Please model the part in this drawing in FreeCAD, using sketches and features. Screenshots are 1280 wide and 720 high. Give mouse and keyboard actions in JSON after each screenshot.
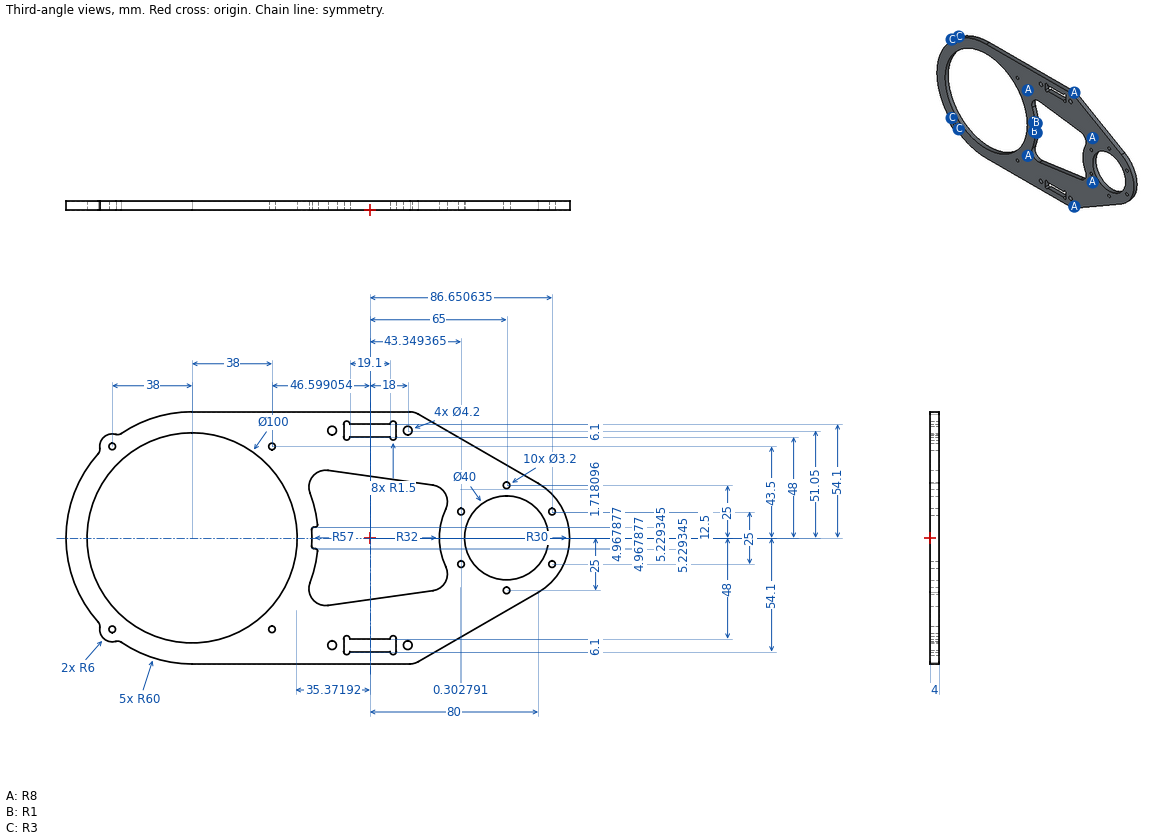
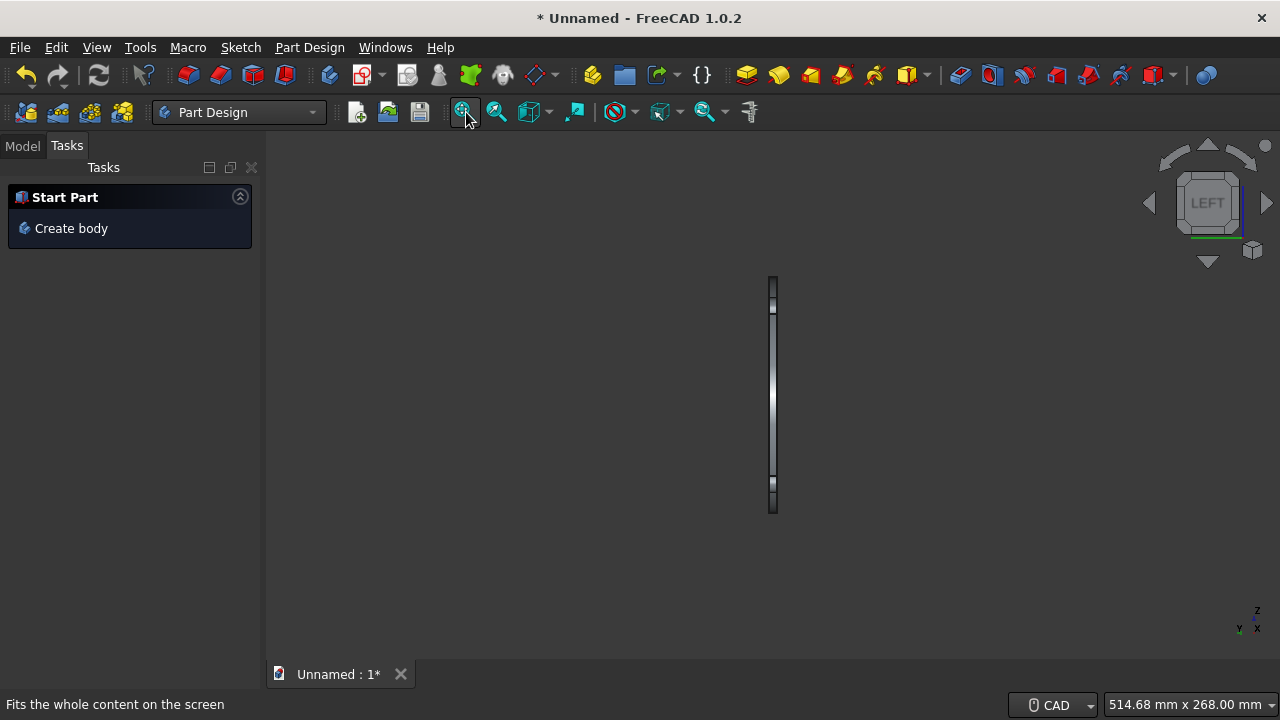
{"action": "scroll", "coordinate": [773, 298], "scroll_direction": "up", "scroll_amount": 9}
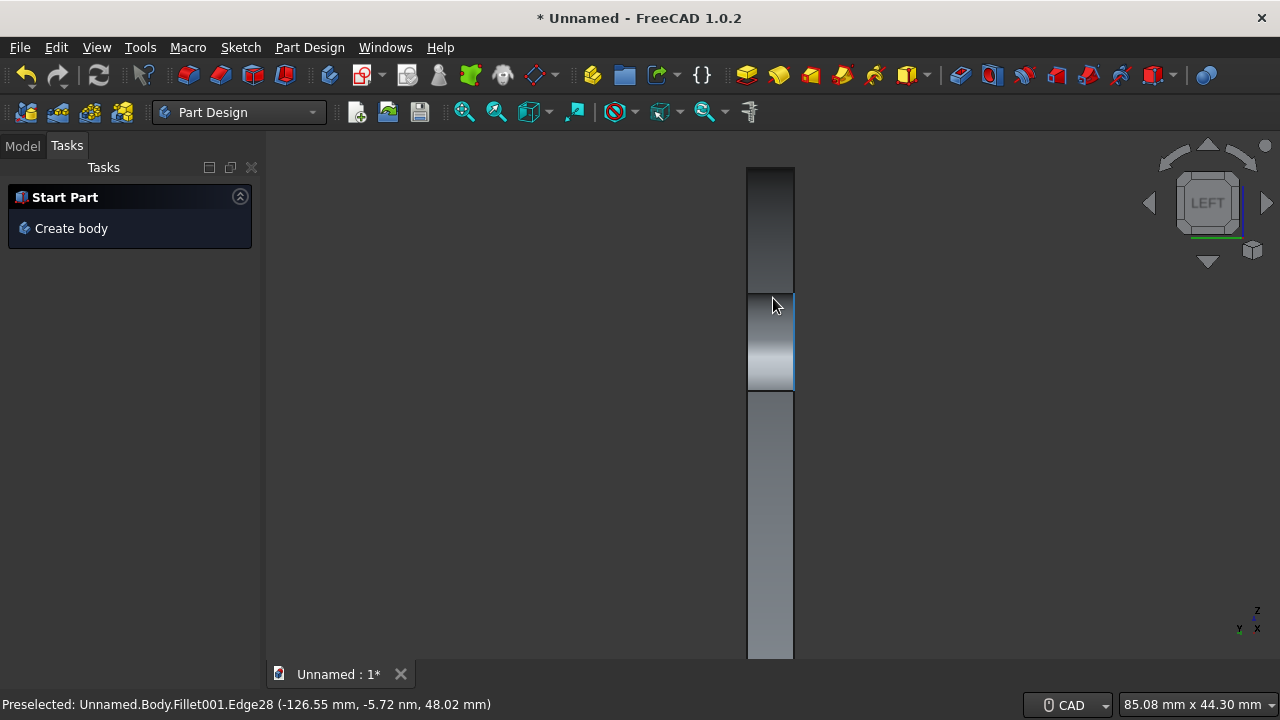
{"action": "key", "text": "v f"}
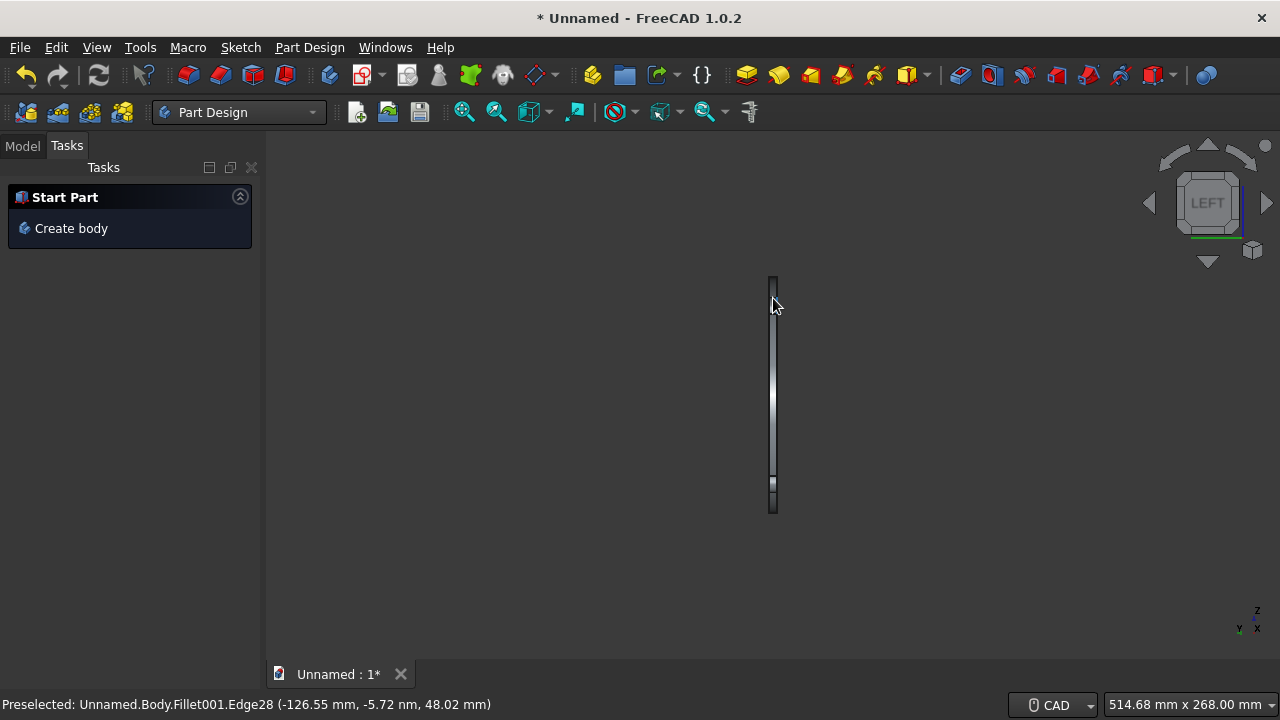
{"action": "key", "text": "v 3"}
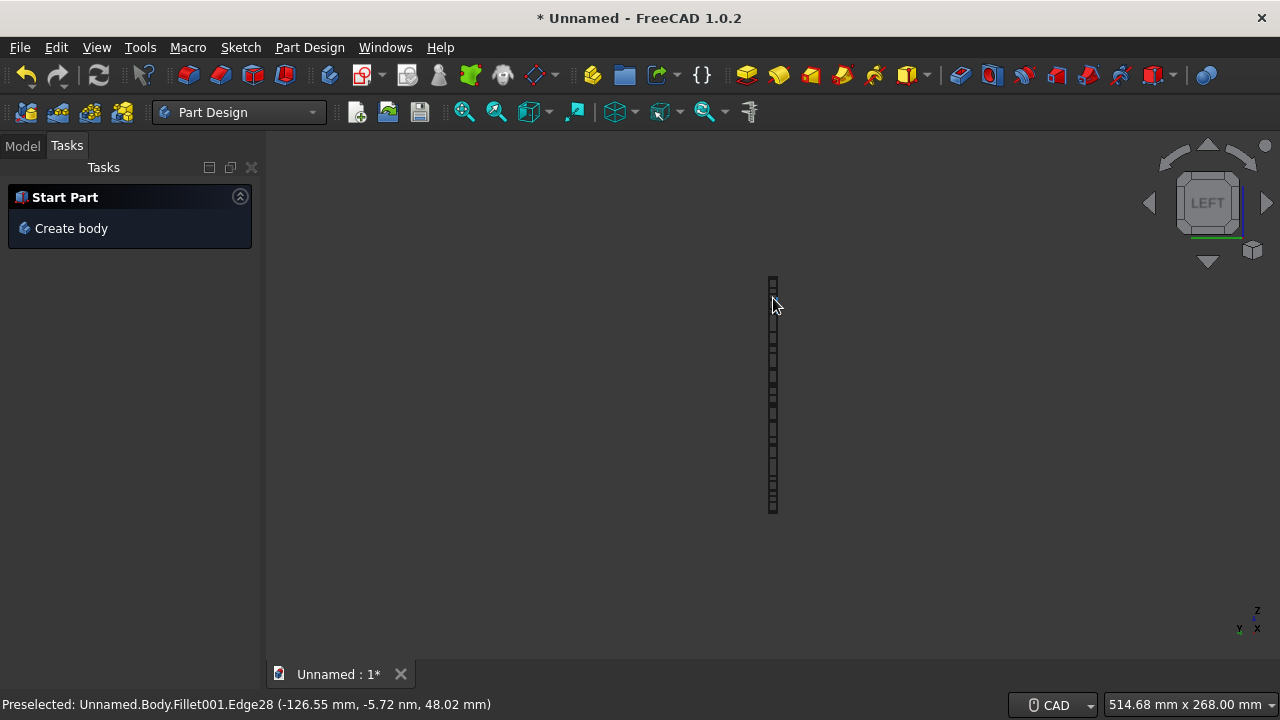
{"action": "key", "text": "0"}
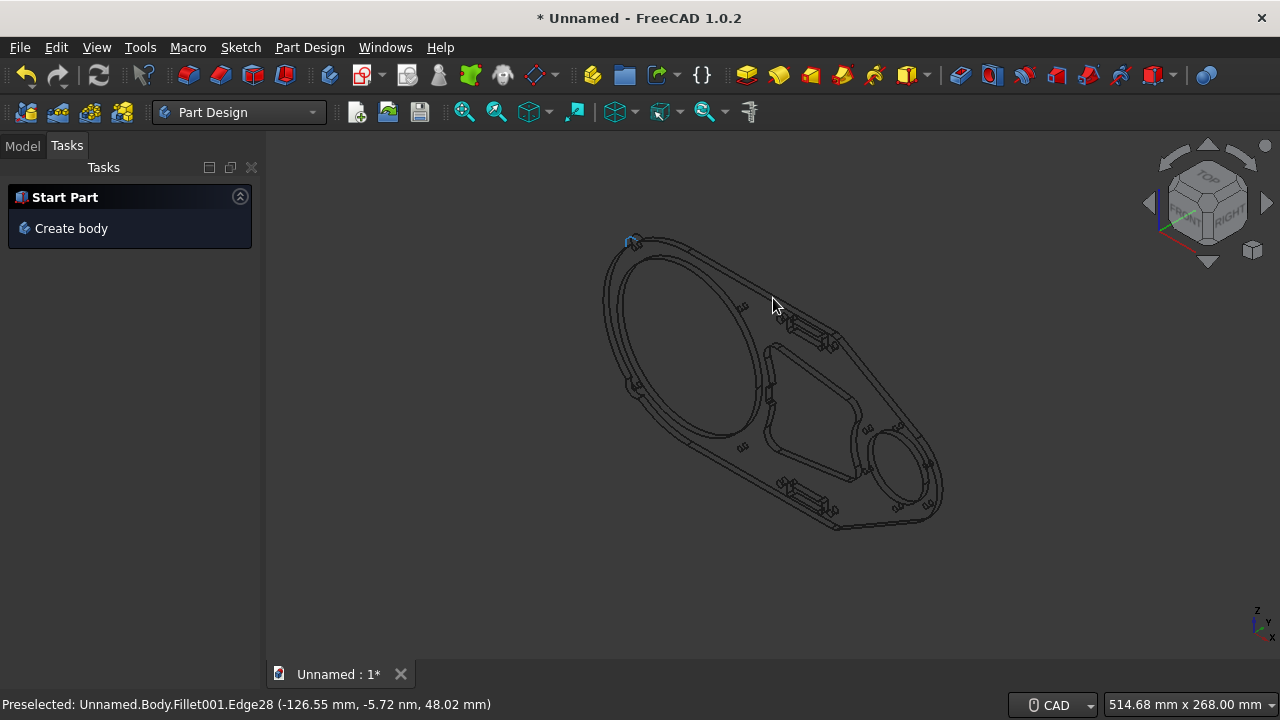
{"action": "scroll", "coordinate": [641, 239], "scroll_direction": "up", "scroll_amount": 9}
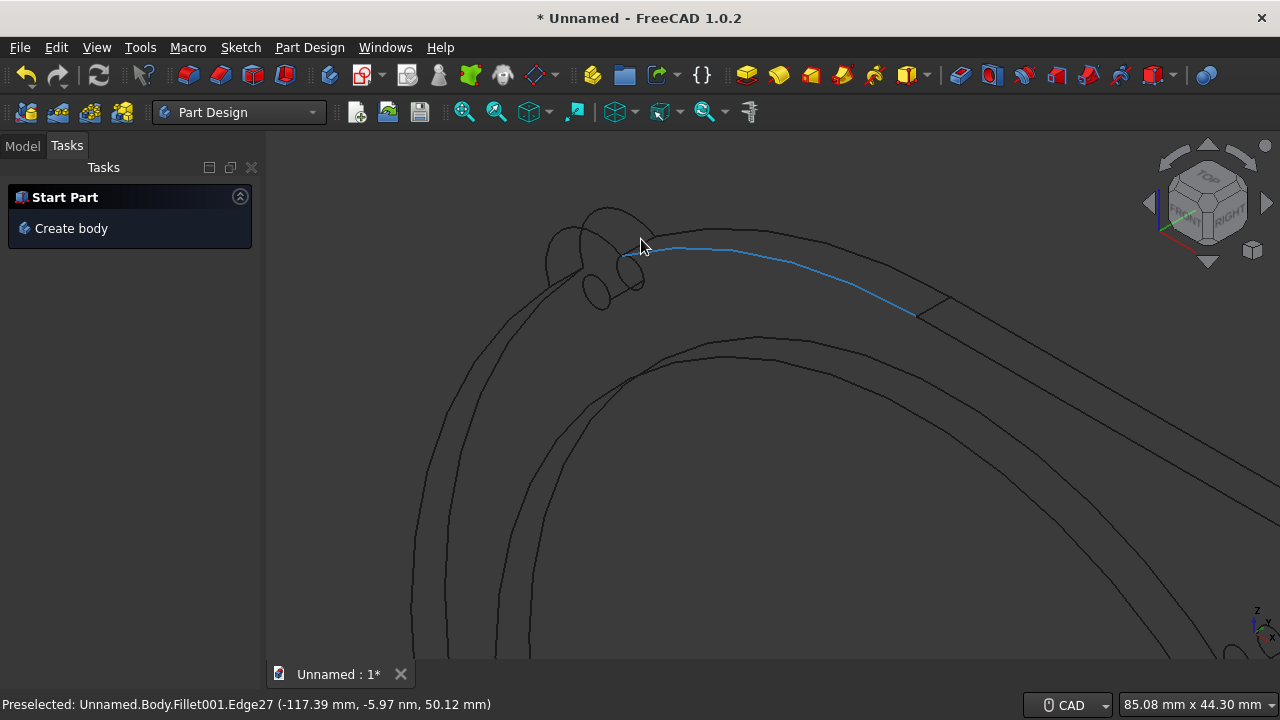
{"action": "left_click", "coordinate": [638, 245]}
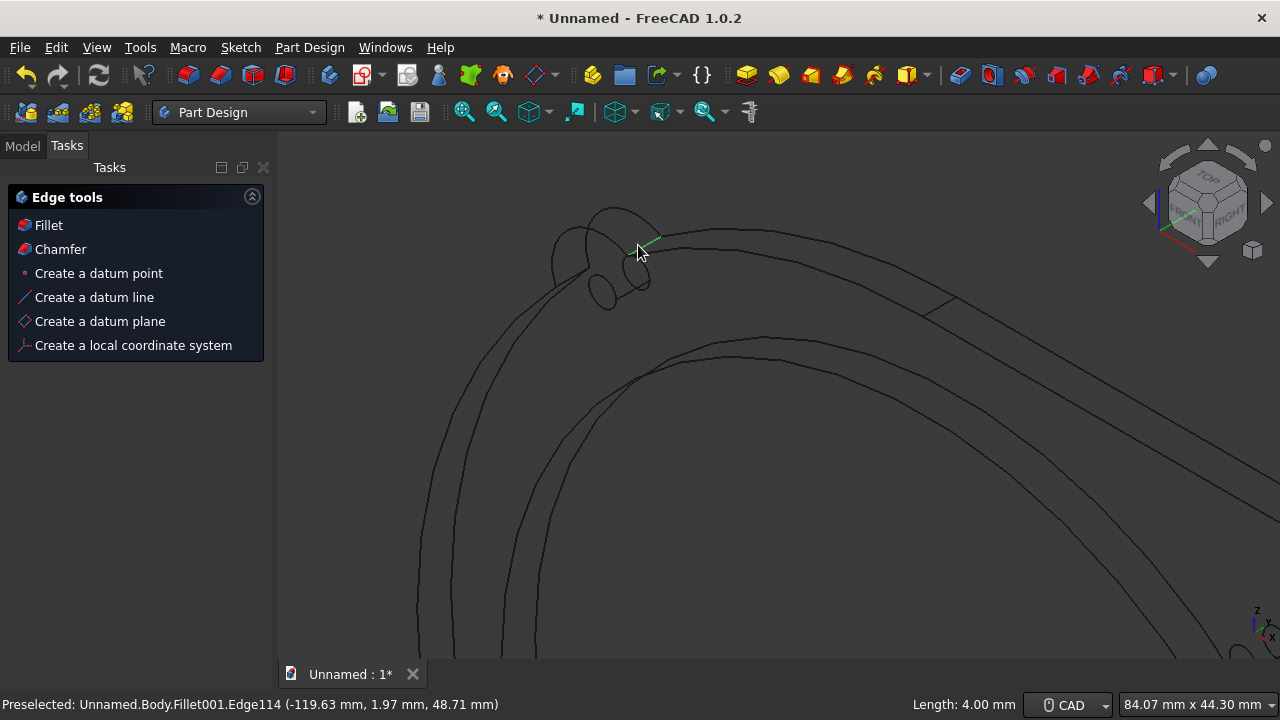
{"action": "left_click", "coordinate": [573, 276], "text": "ctrl"}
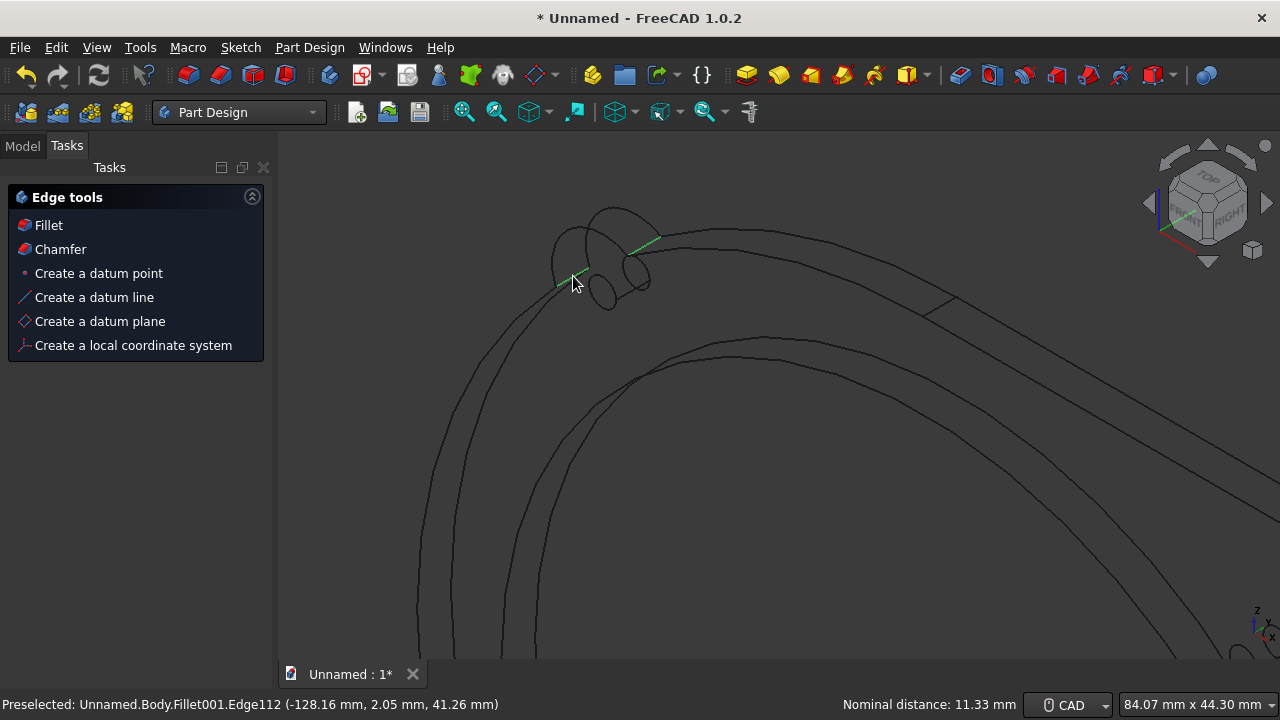
{"action": "left_click", "coordinate": [466, 112]}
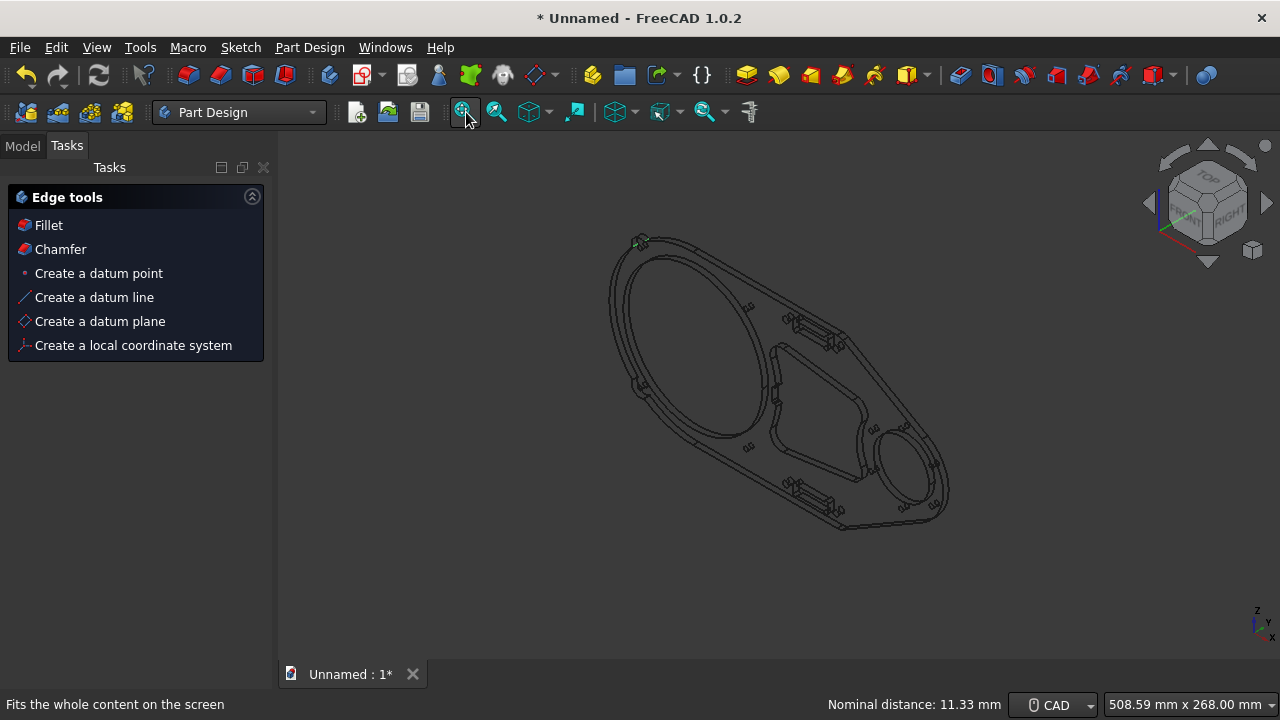
{"action": "key", "text": "2"}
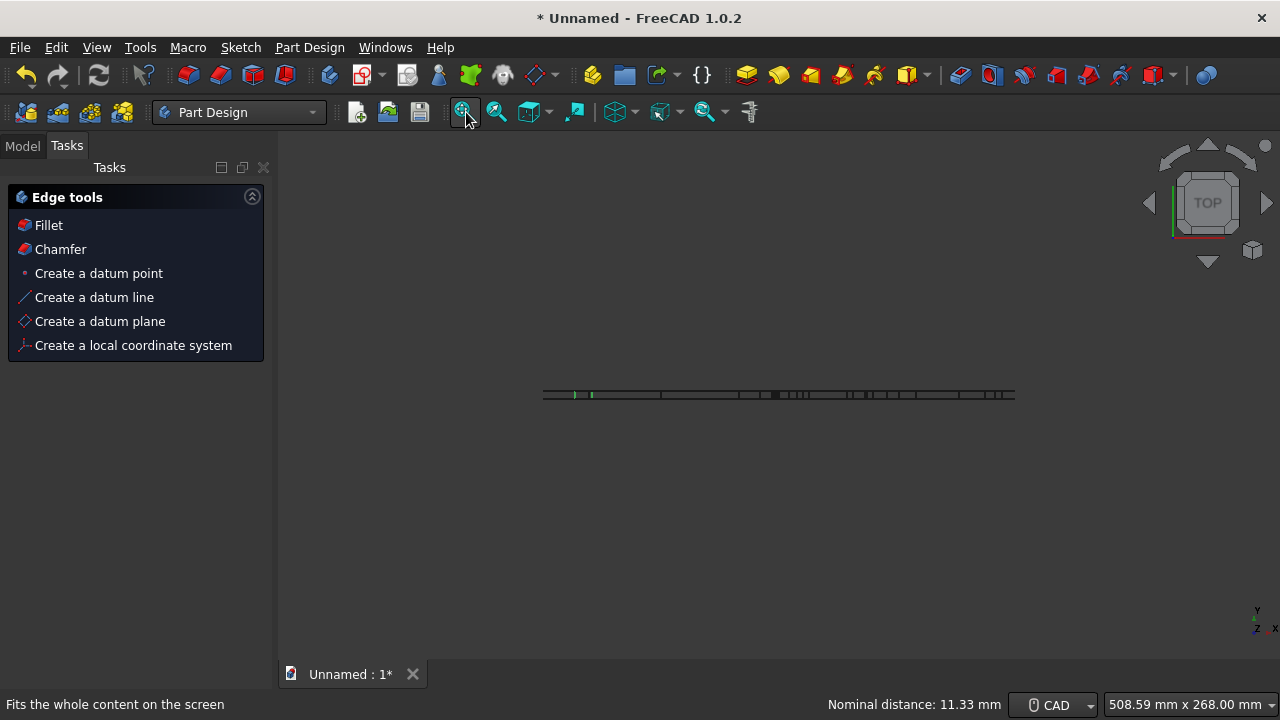
{"action": "scroll", "coordinate": [575, 394], "scroll_direction": "up", "scroll_amount": 9}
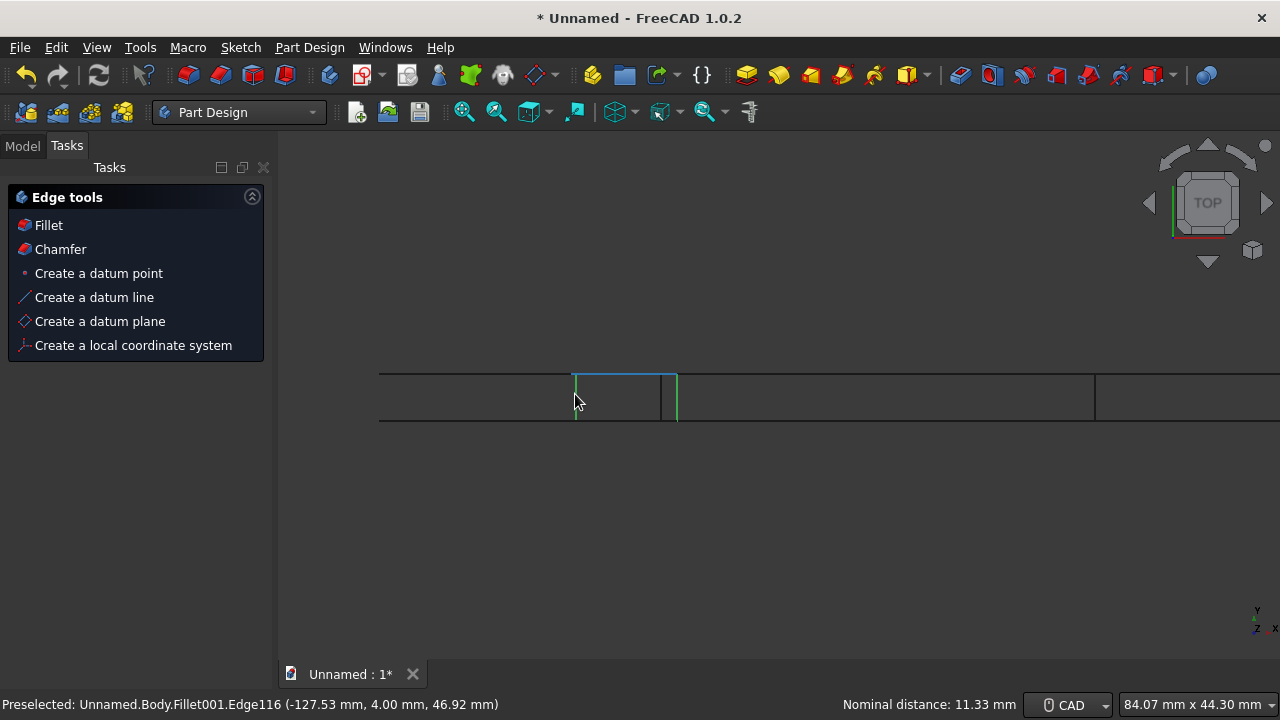
{"action": "left_click", "coordinate": [466, 112]}